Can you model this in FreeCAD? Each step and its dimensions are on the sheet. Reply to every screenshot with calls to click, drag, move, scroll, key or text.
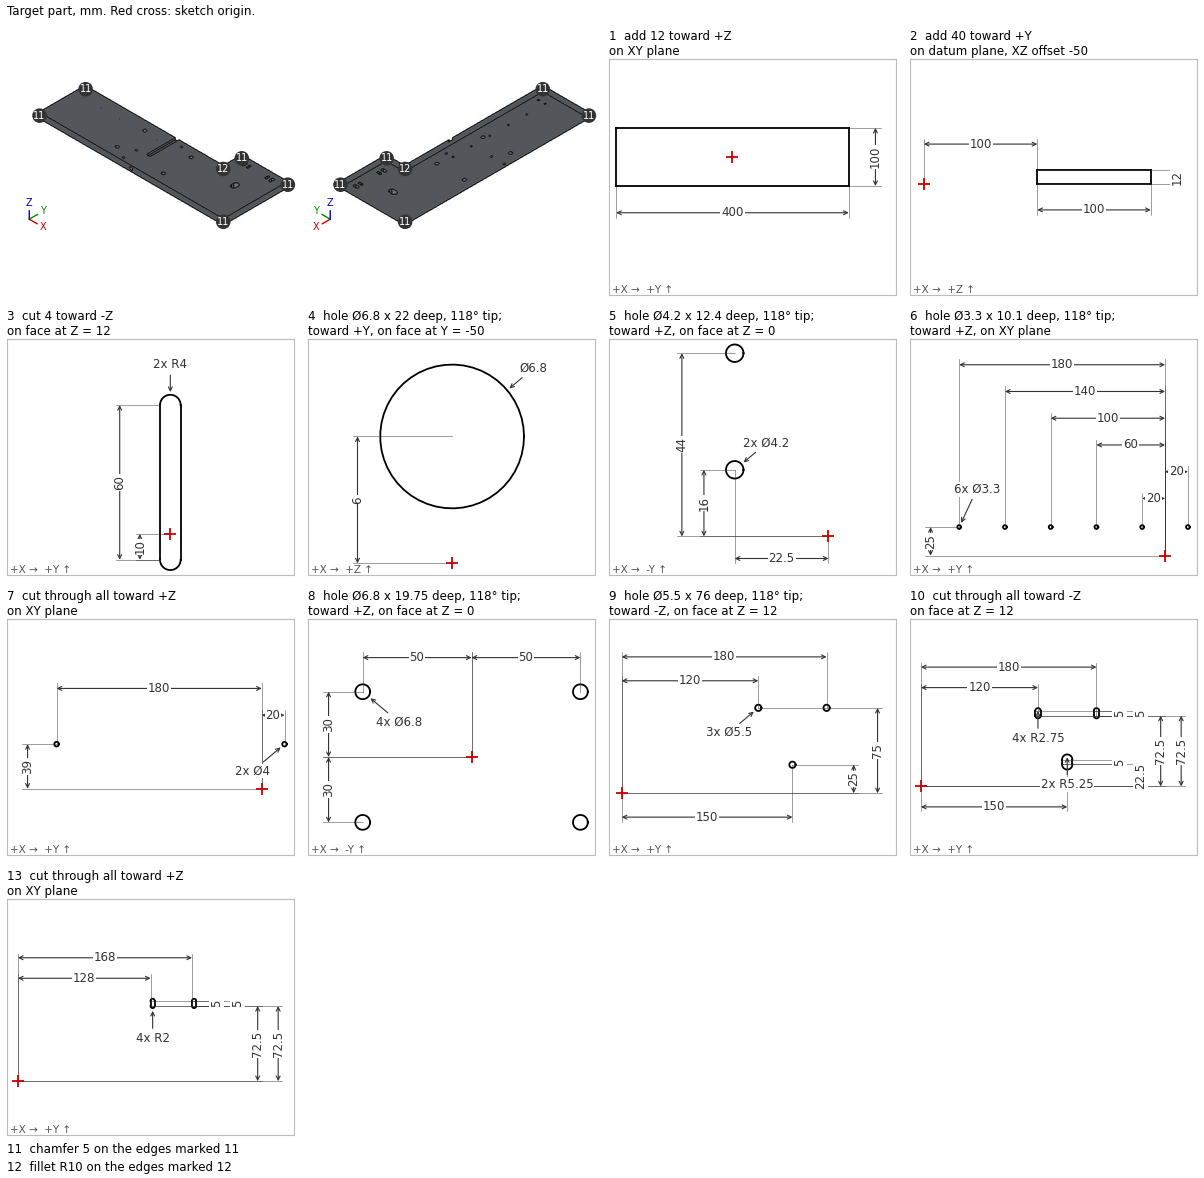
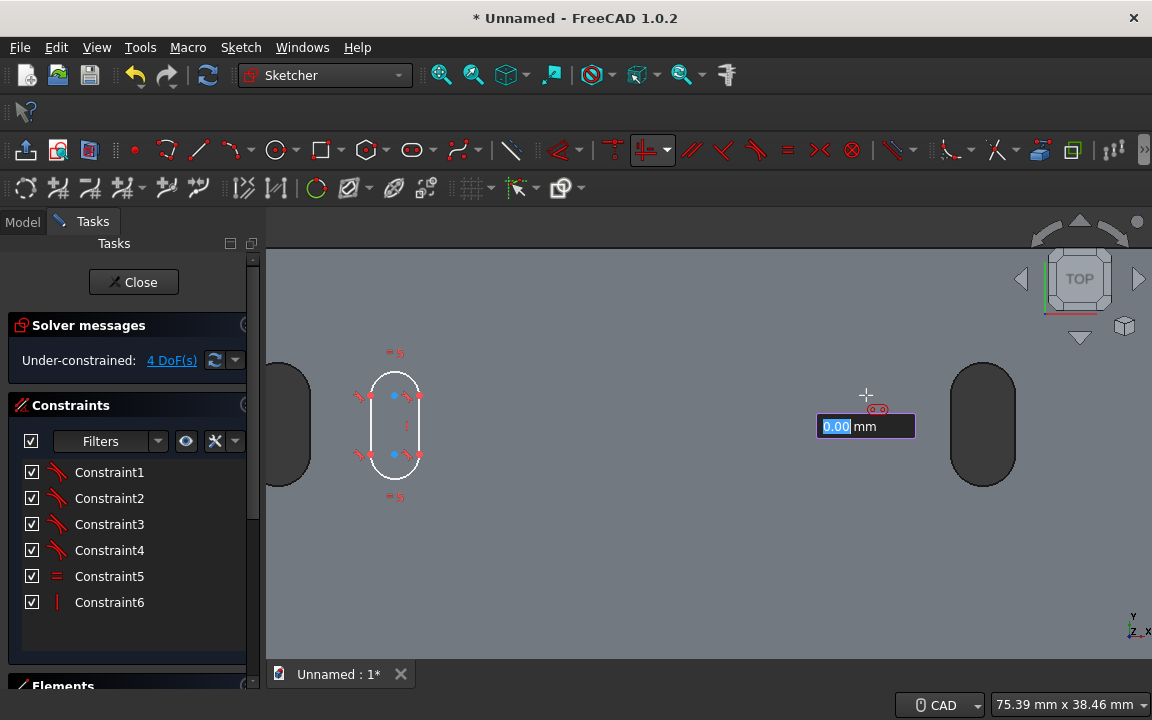
click(889, 425)
key(Escape)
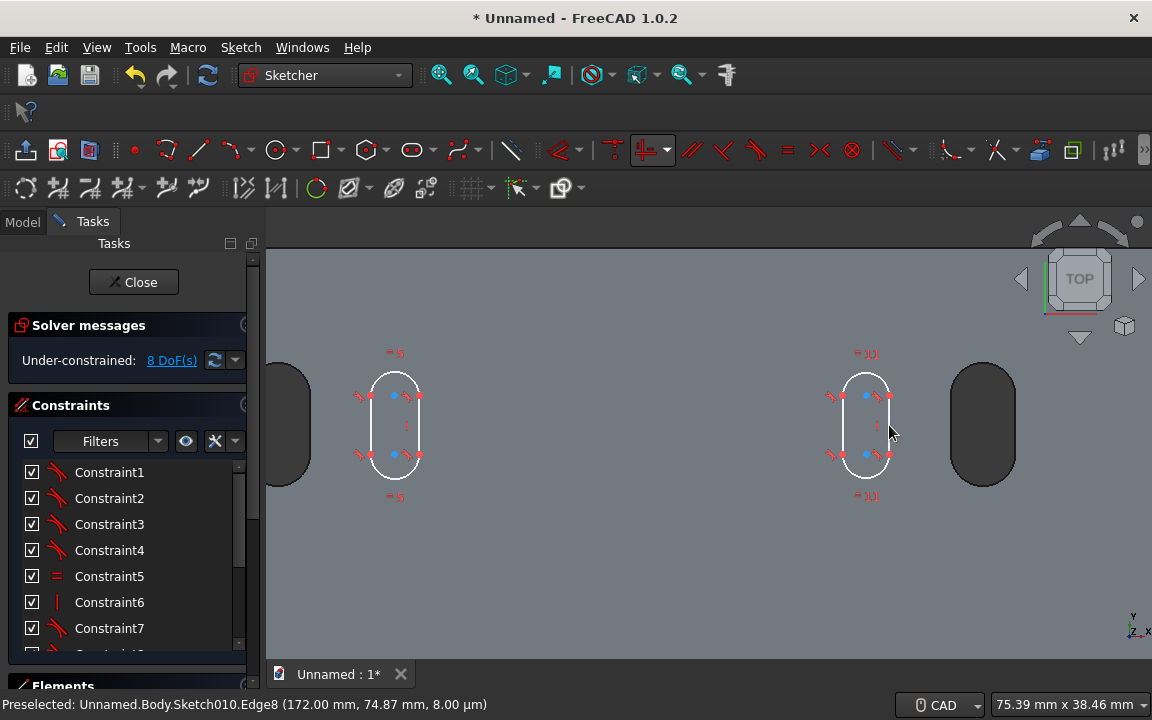
click(381, 474)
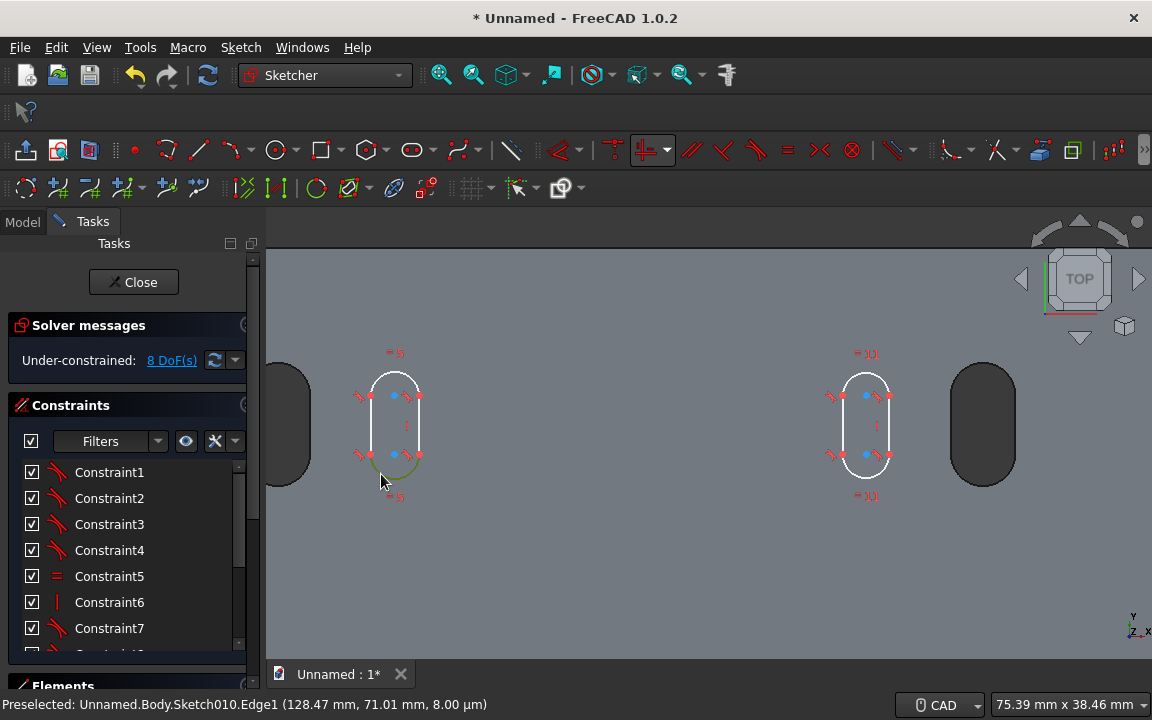
click(852, 474)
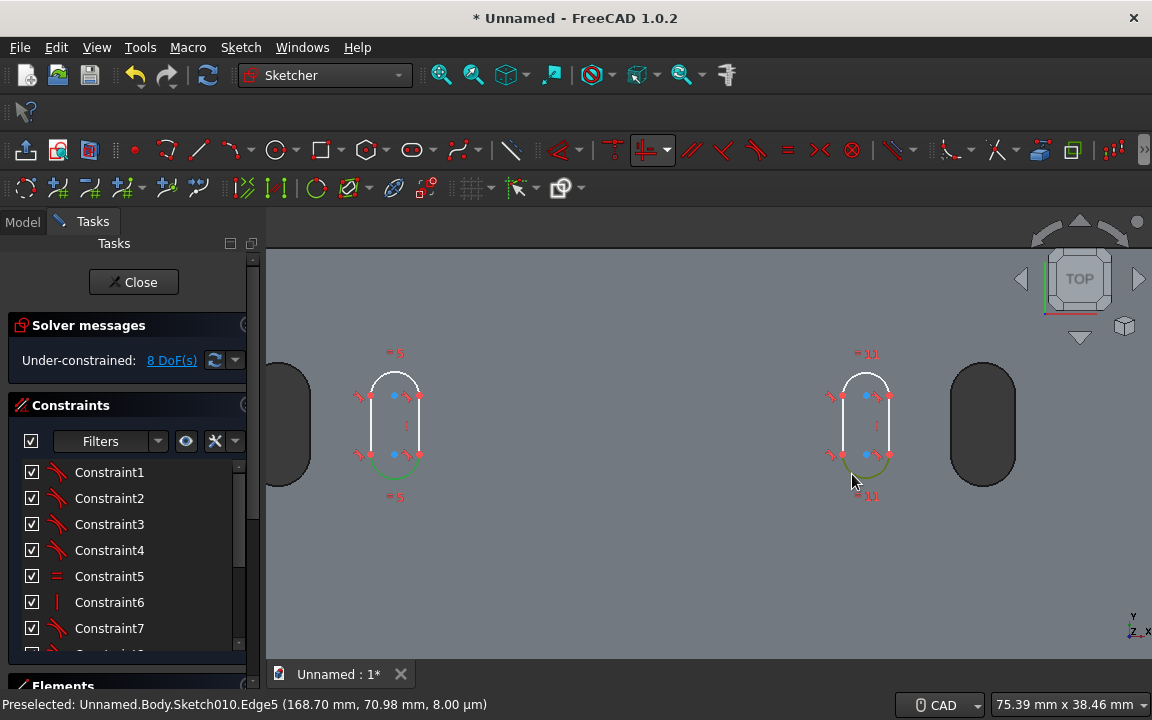
click(788, 150)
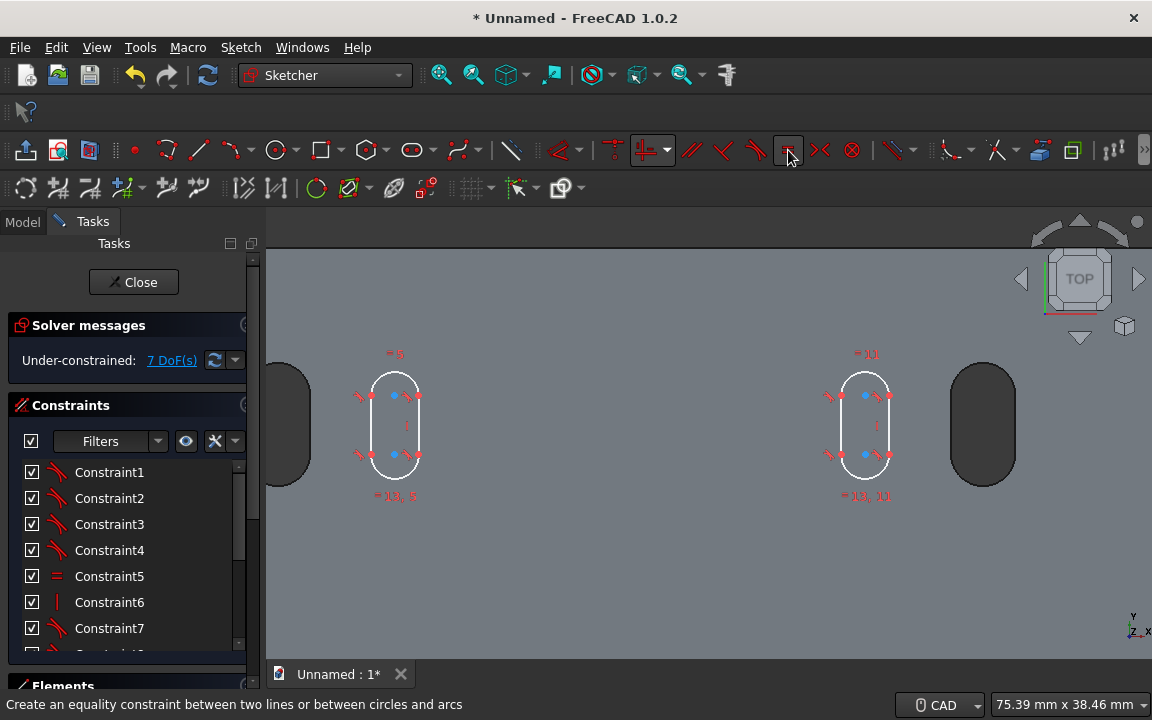
click(558, 150)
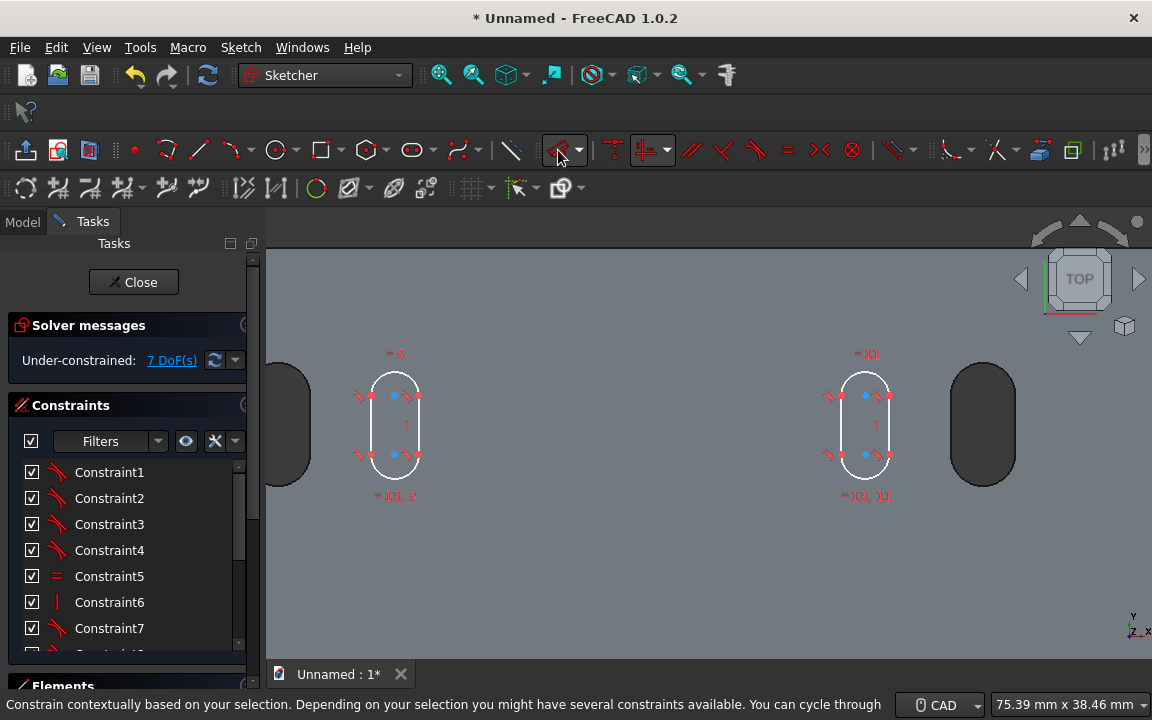
scroll(381, 474, up, 3)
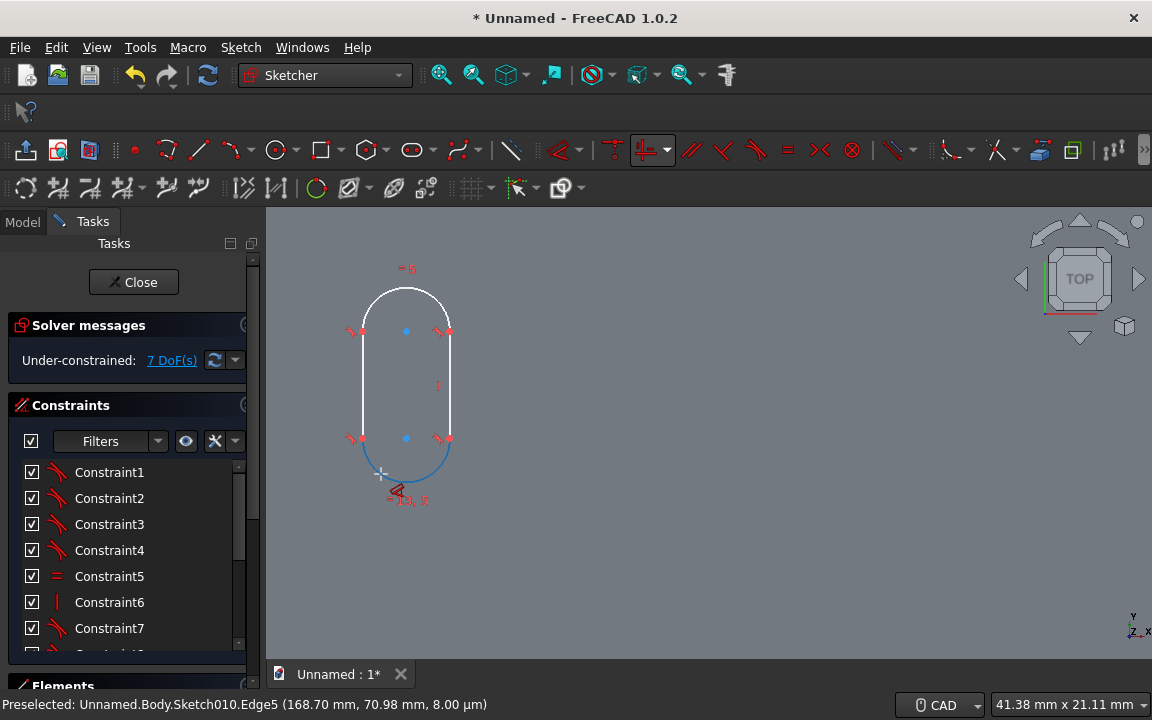
click(381, 474)
click(362, 500)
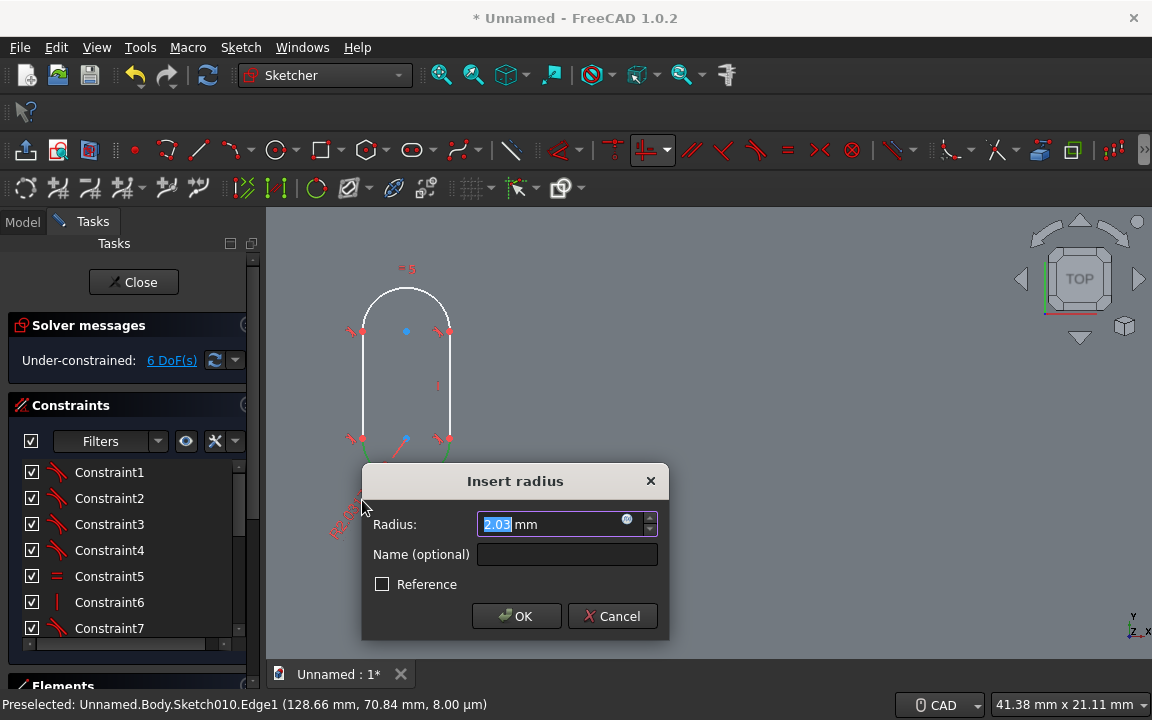
text(2)
key(Return)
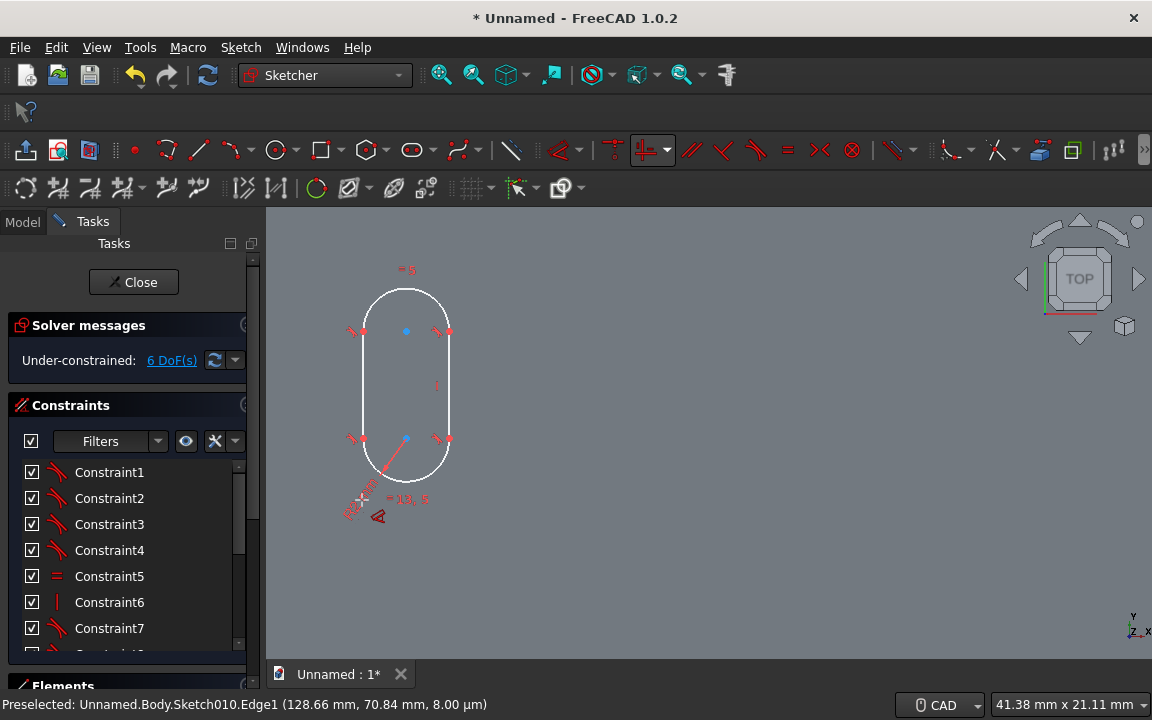
click(364, 407)
click(330, 385)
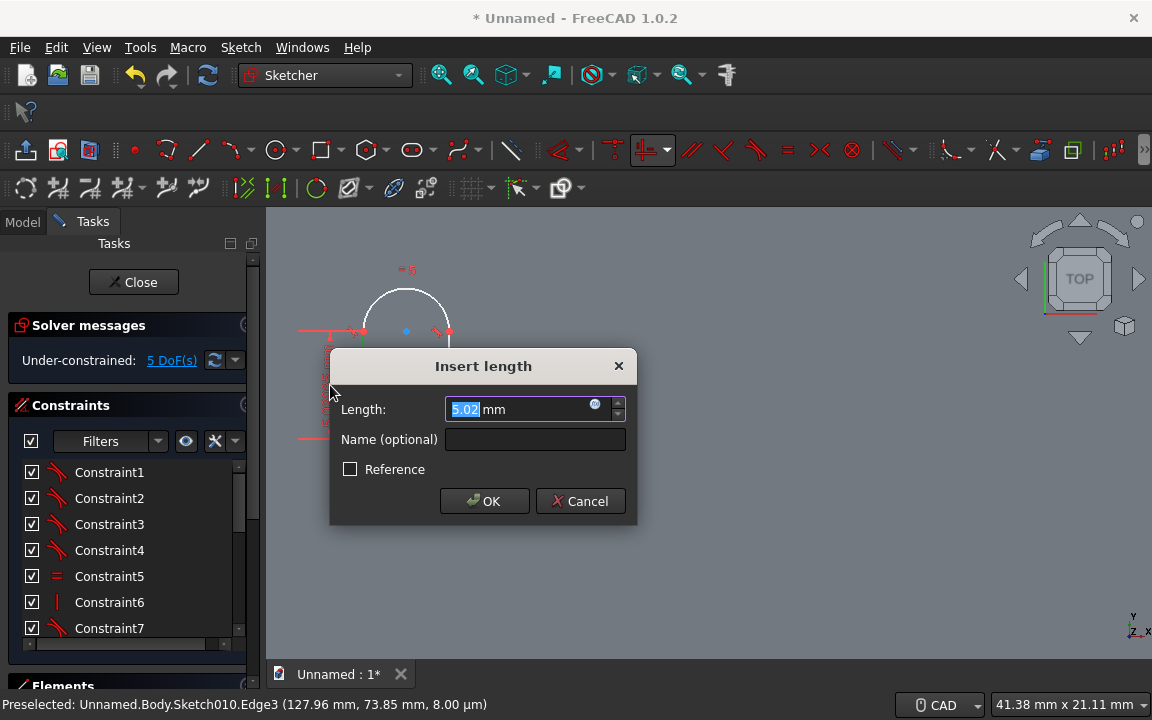
text(5)
key(Return)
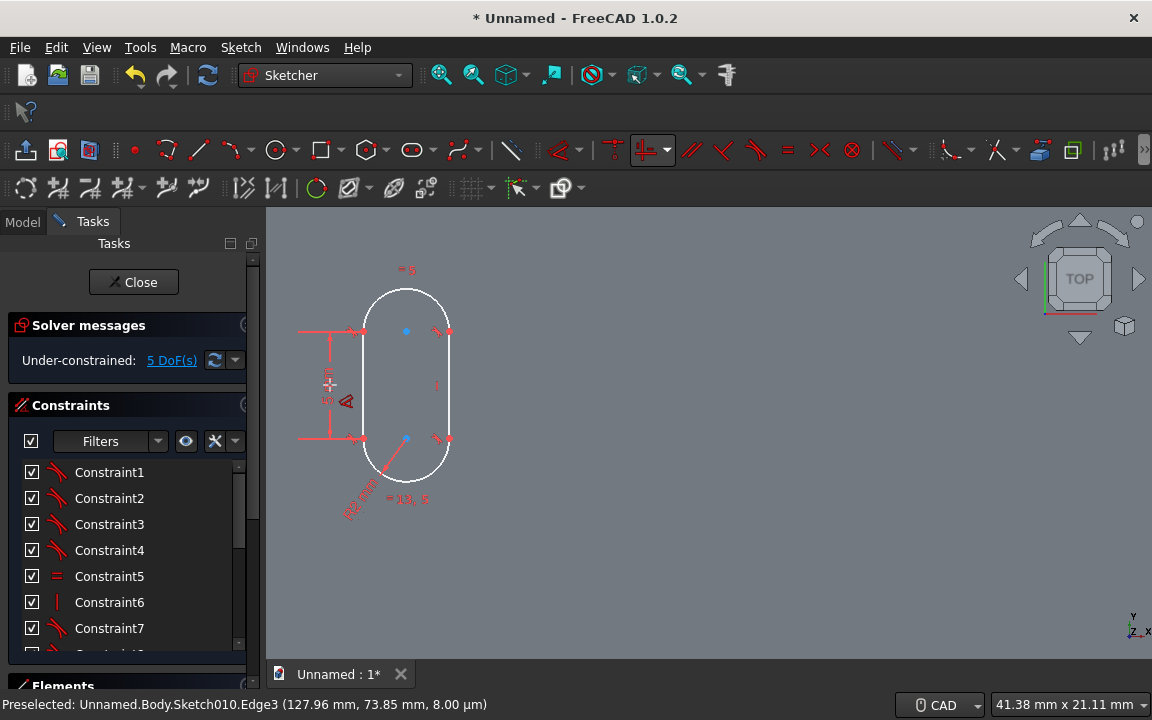
scroll(403, 493, down, 3)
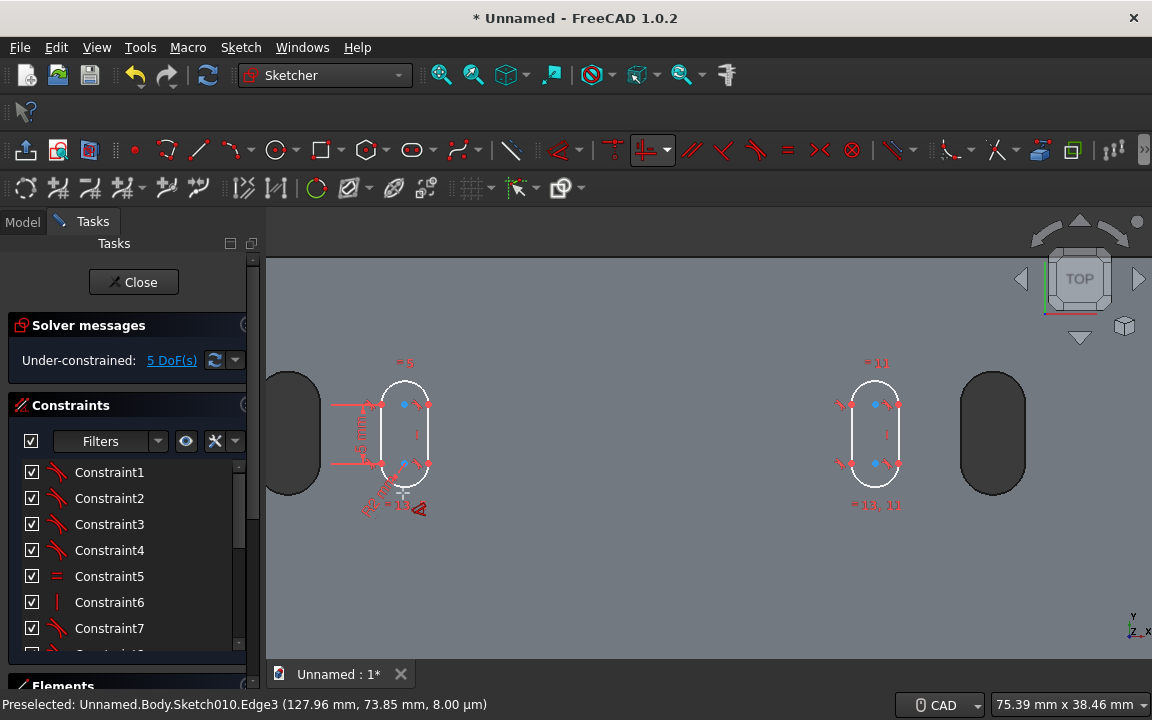
click(852, 446)
click(886, 434)